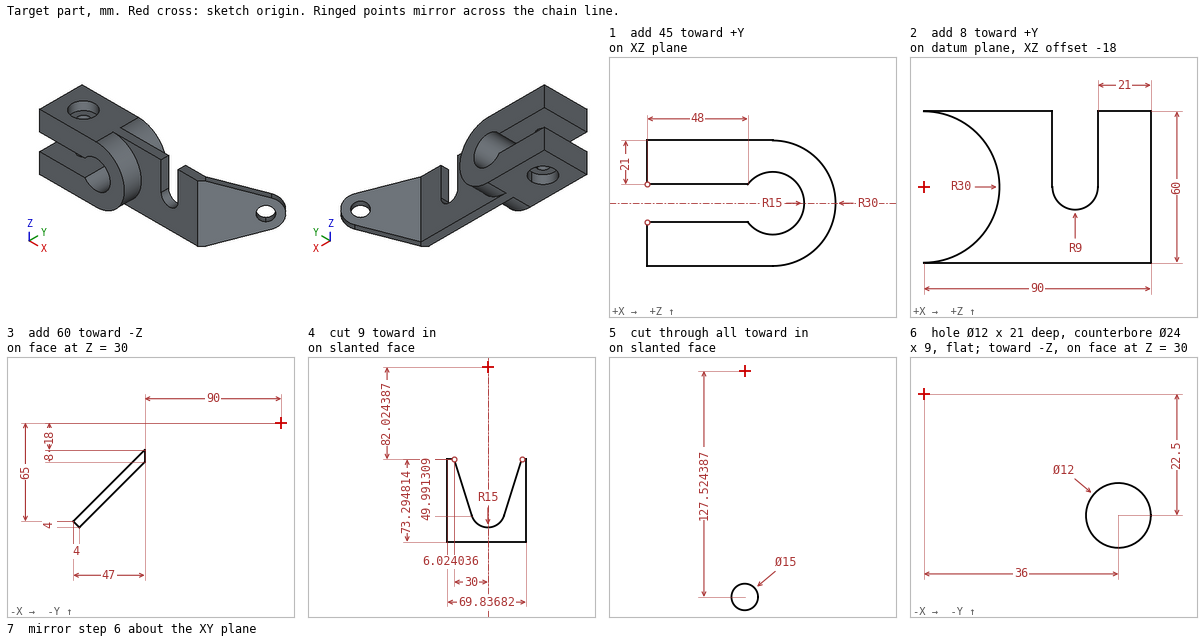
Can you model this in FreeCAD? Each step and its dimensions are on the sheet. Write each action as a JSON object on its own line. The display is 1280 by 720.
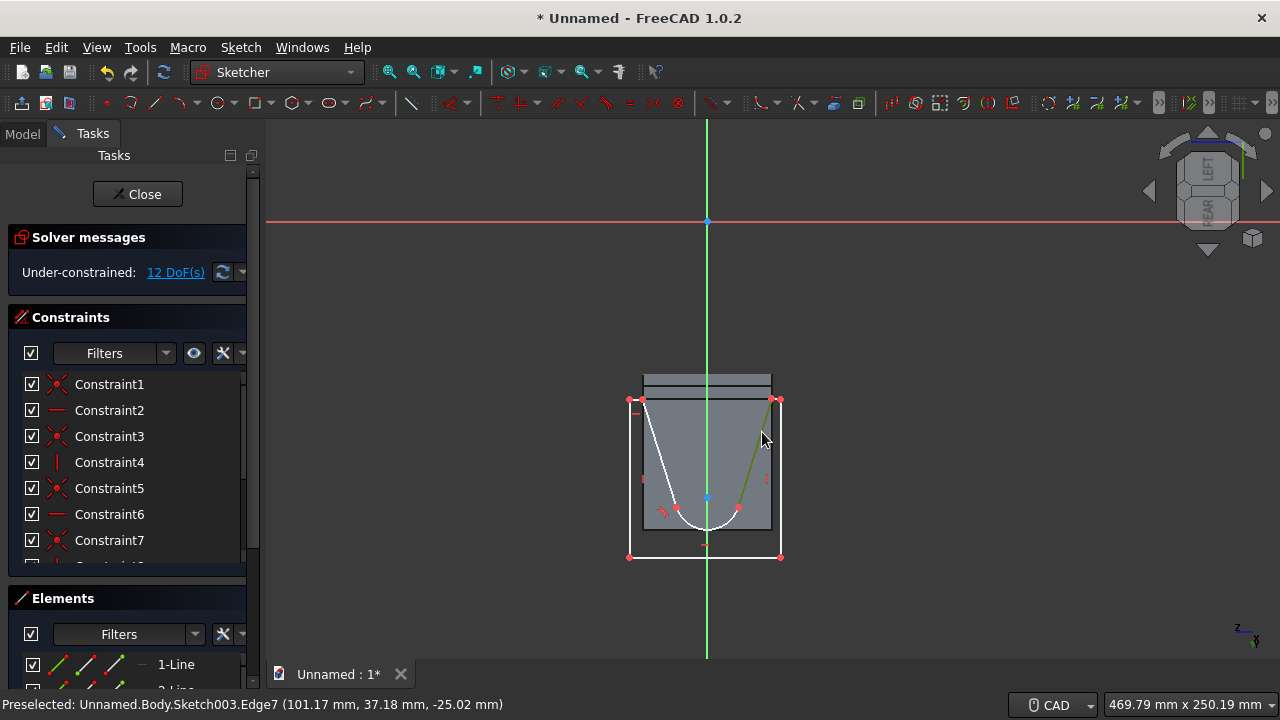
{"action": "left_click", "coordinate": [692, 526]}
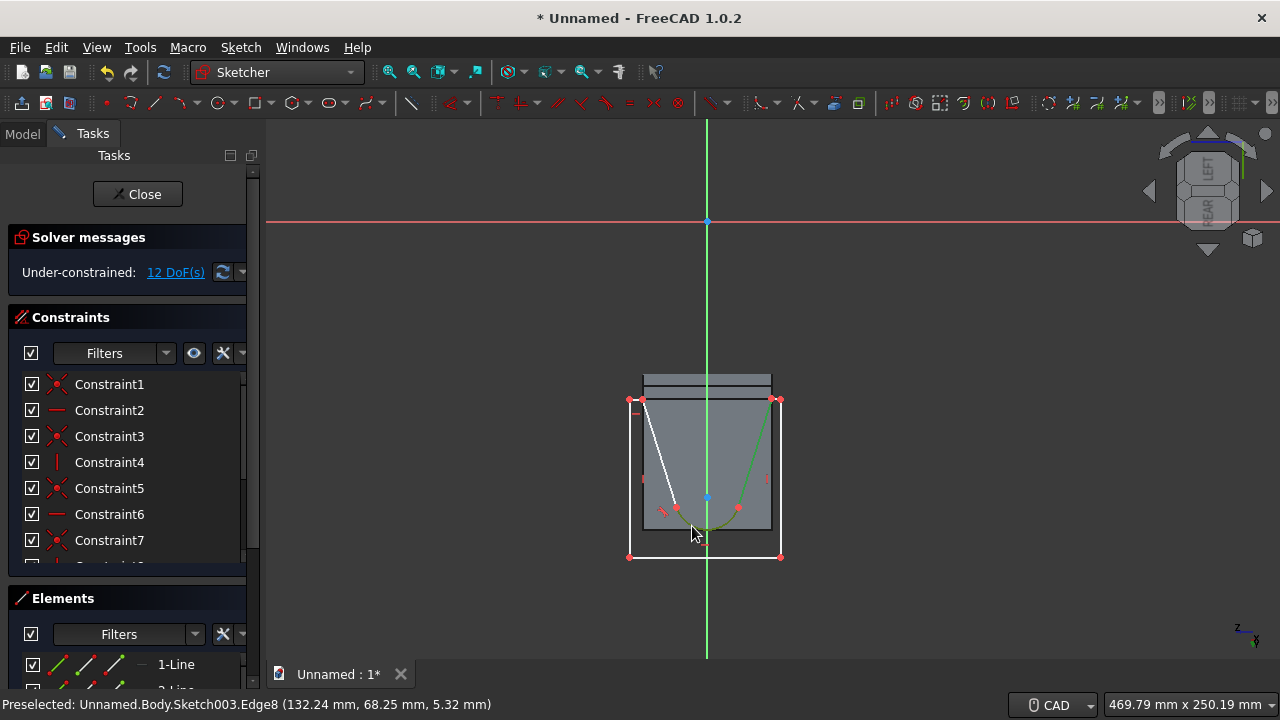
{"action": "key", "text": "t"}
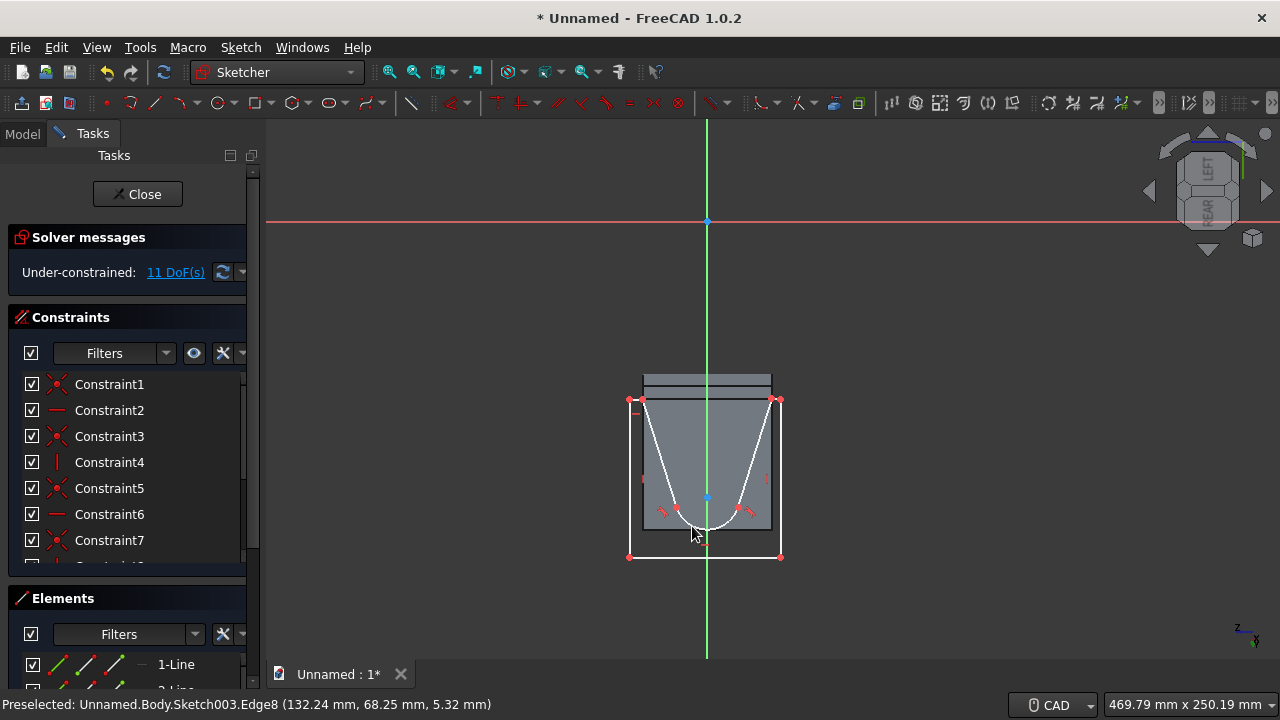
{"action": "scroll", "coordinate": [776, 399], "scroll_direction": "up", "scroll_amount": 6}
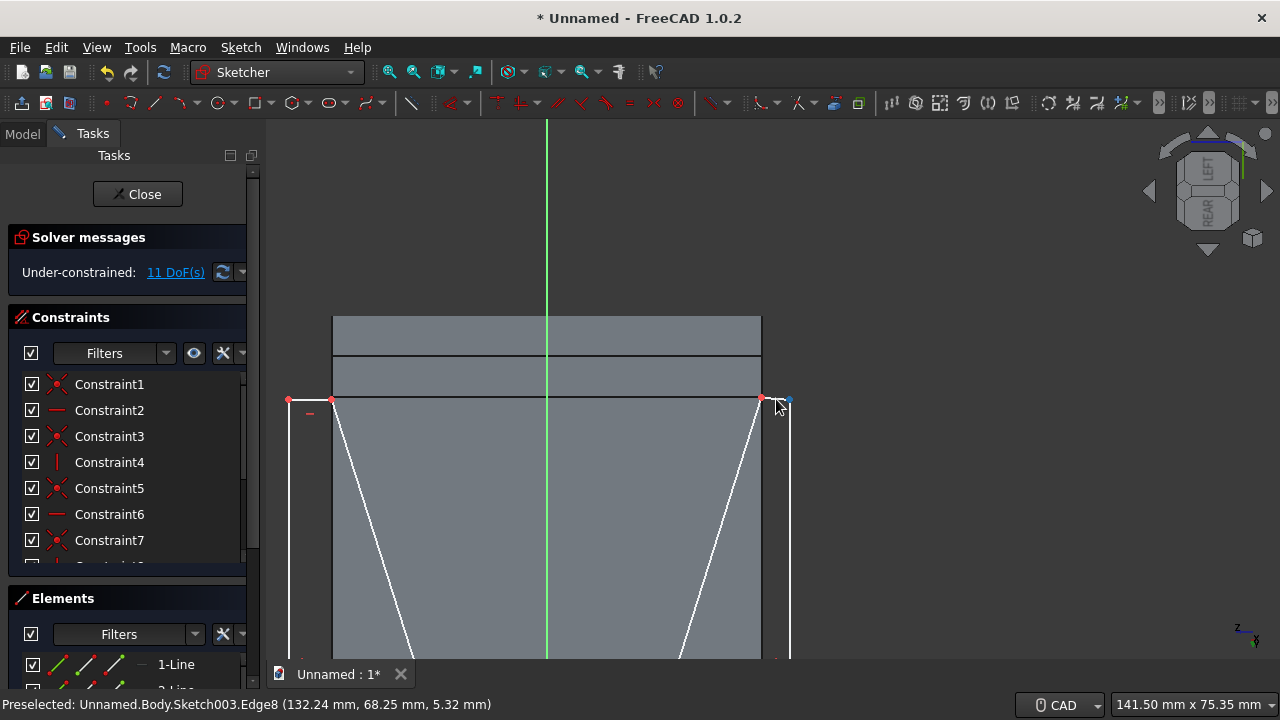
{"action": "left_click", "coordinate": [776, 399]}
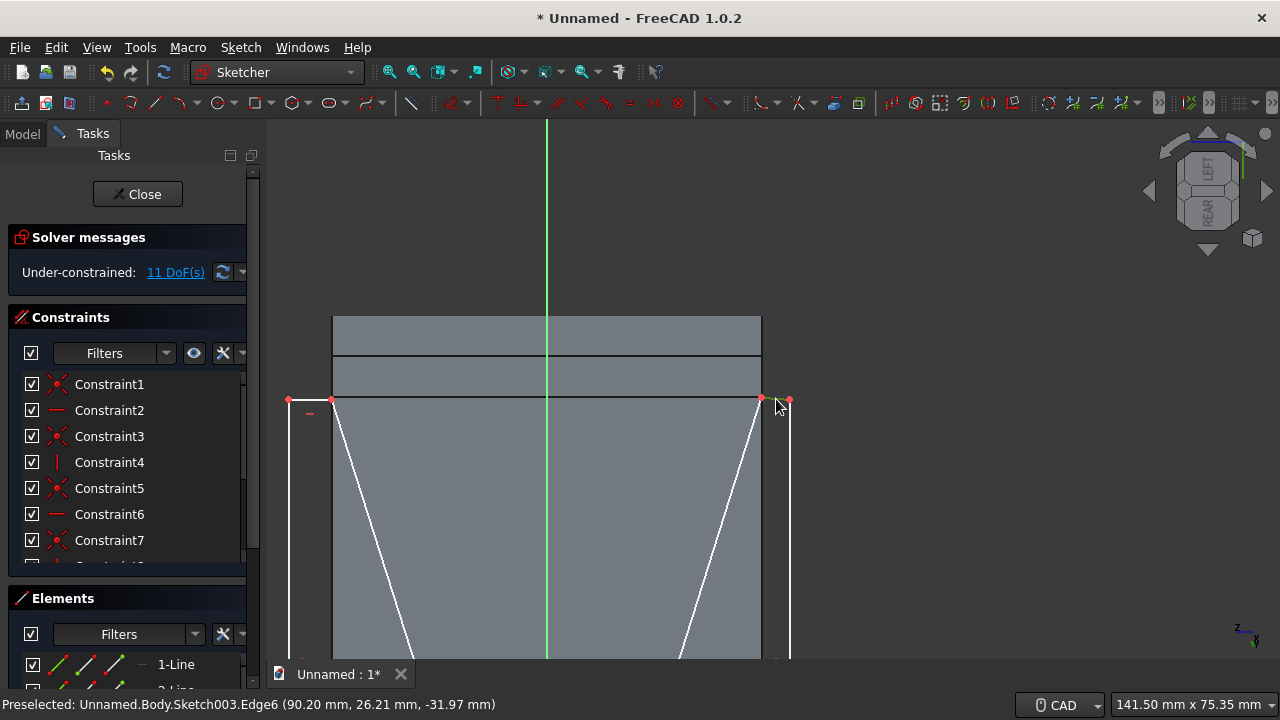
{"action": "left_click", "coordinate": [540, 104]}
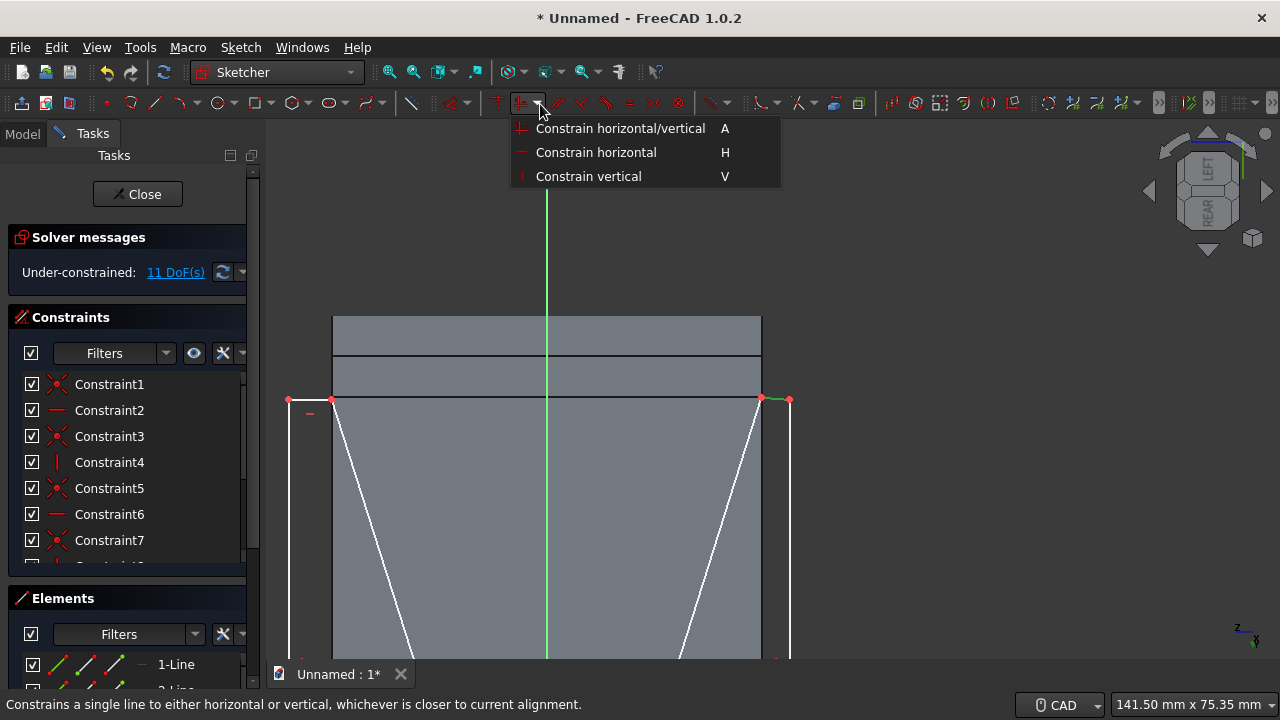
{"action": "left_click", "coordinate": [646, 152]}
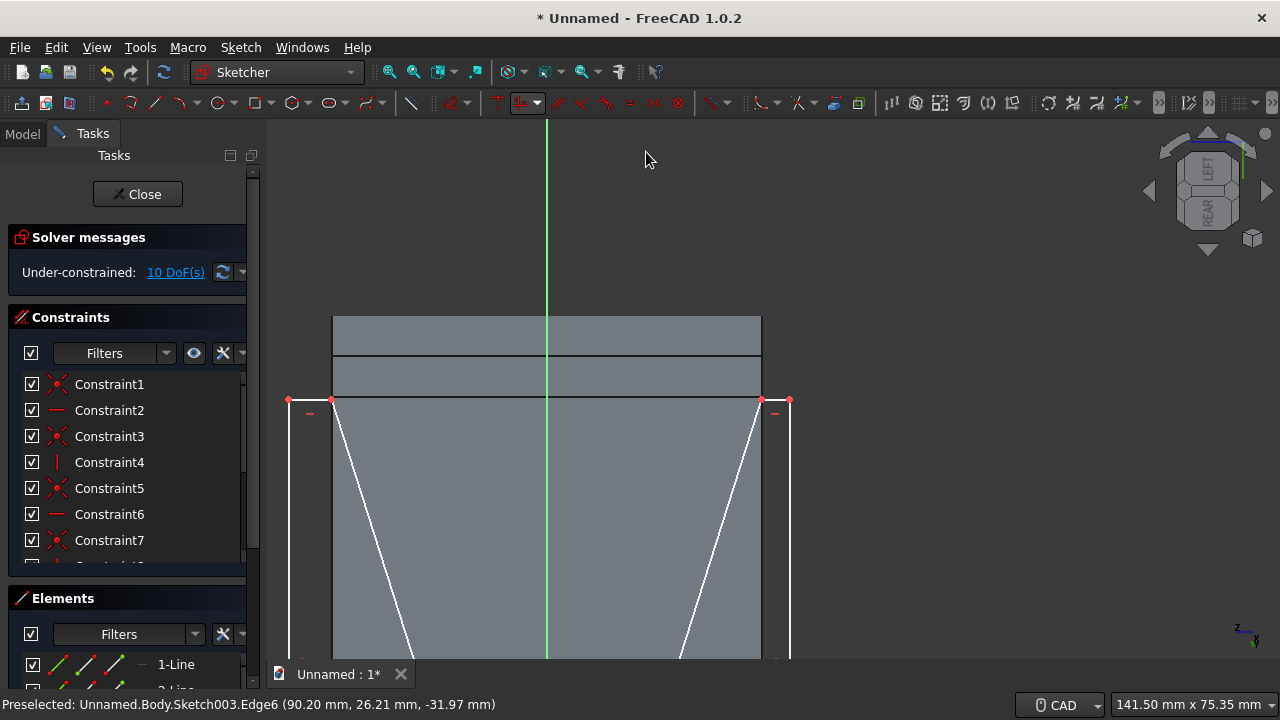
{"action": "scroll", "coordinate": [776, 399], "scroll_direction": "down", "scroll_amount": 6}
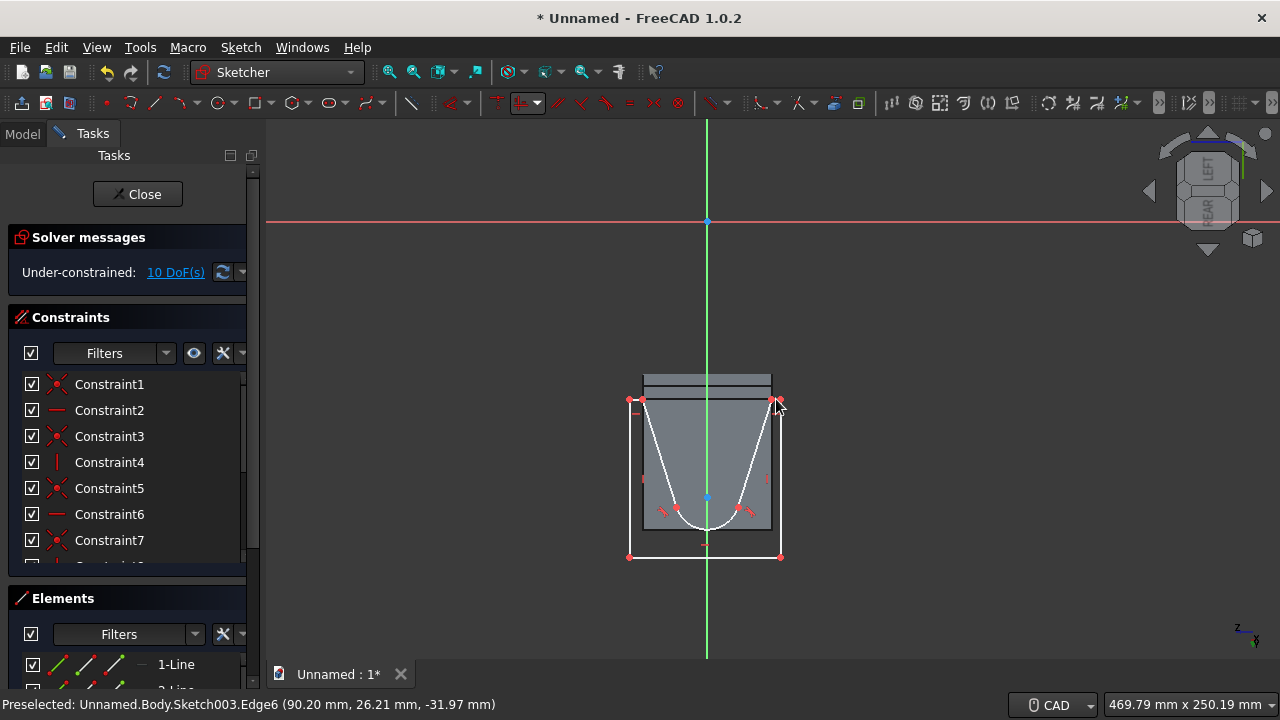
{"action": "left_click", "coordinate": [707, 497]}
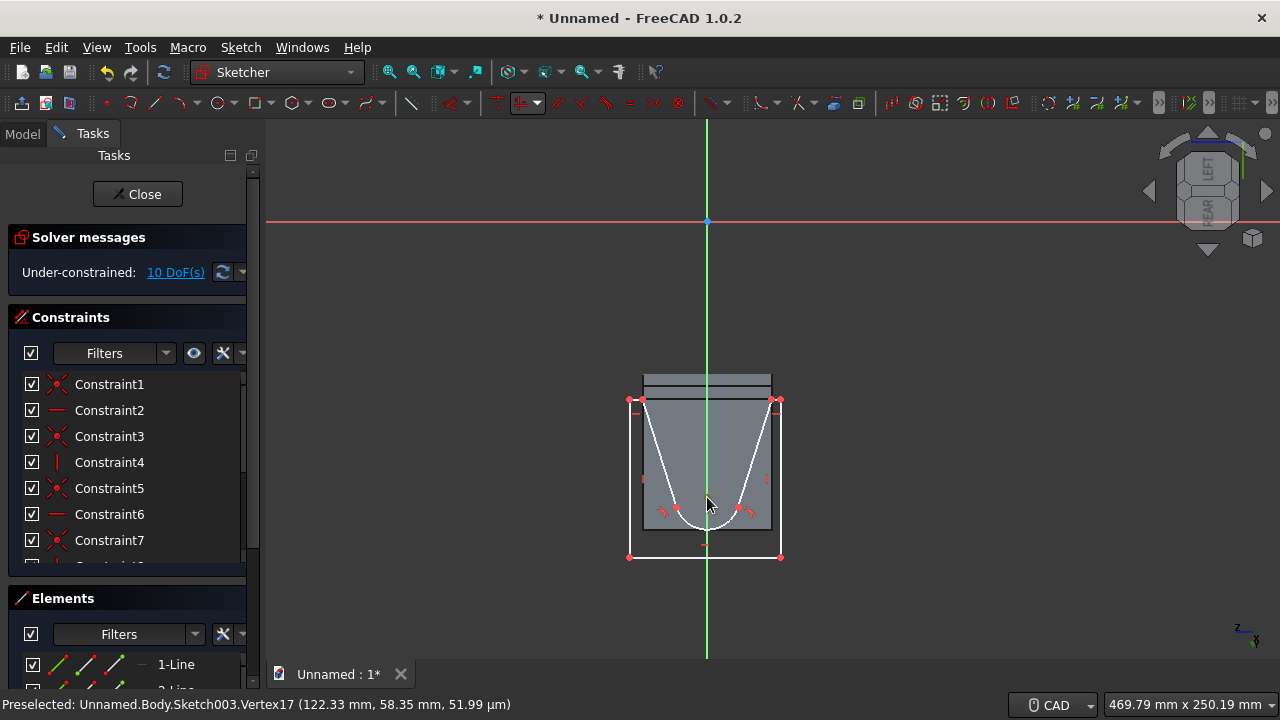
{"action": "left_click", "coordinate": [707, 596]}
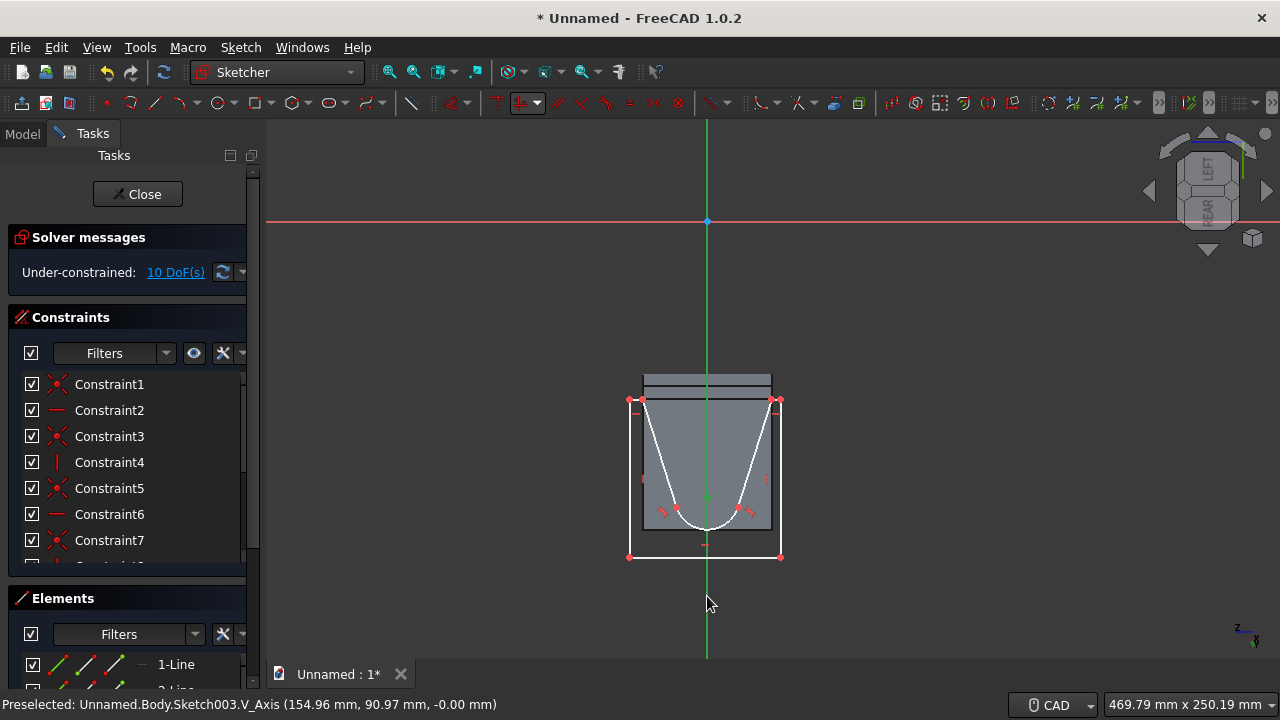
{"action": "left_click", "coordinate": [498, 104]}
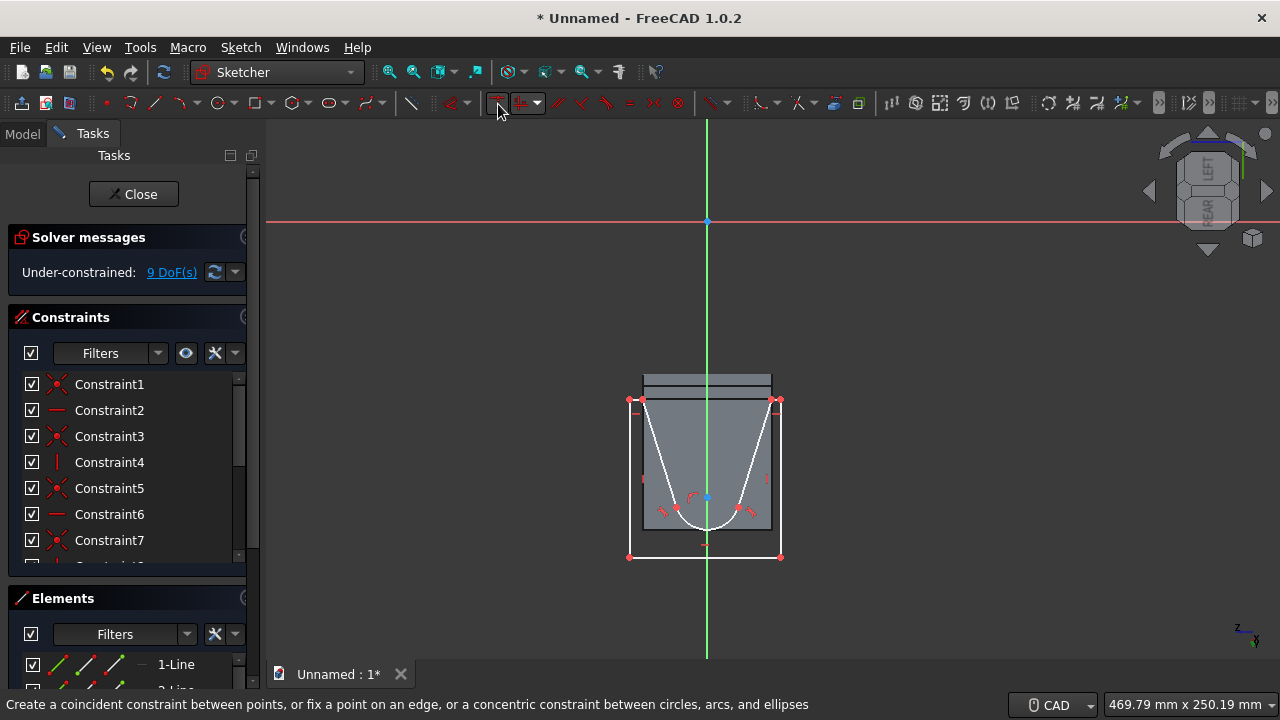
{"action": "left_click", "coordinate": [643, 400]}